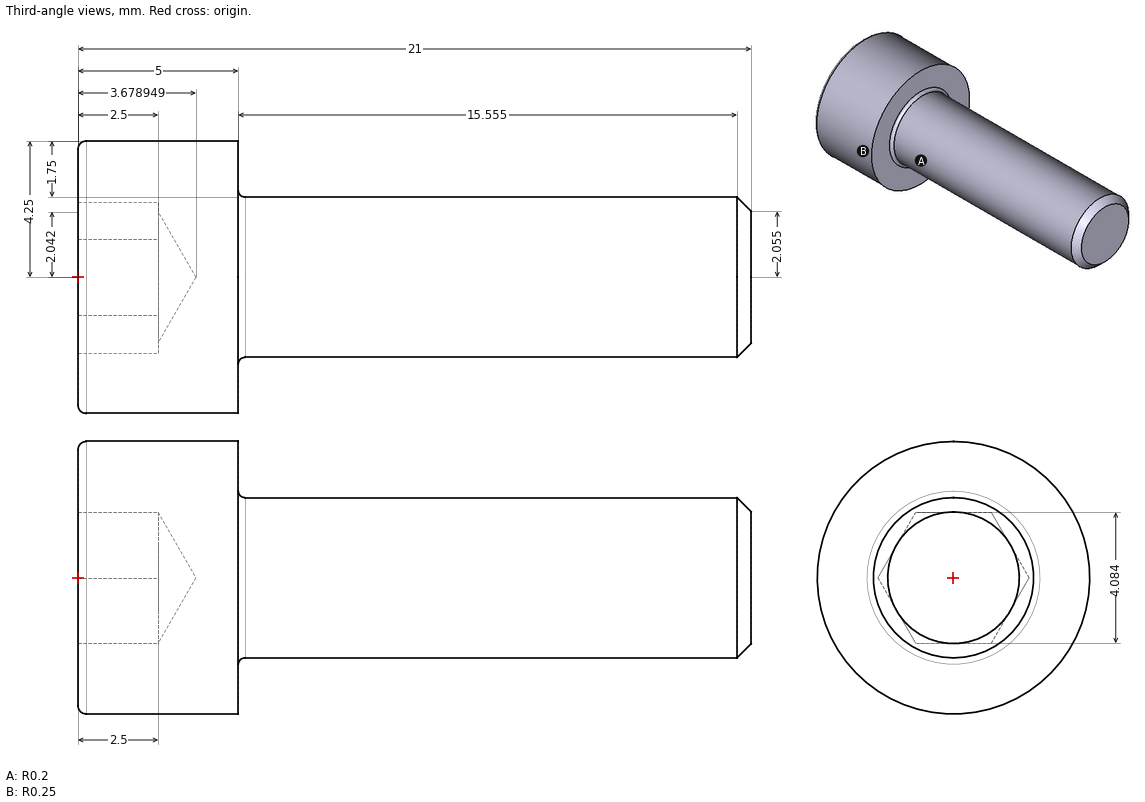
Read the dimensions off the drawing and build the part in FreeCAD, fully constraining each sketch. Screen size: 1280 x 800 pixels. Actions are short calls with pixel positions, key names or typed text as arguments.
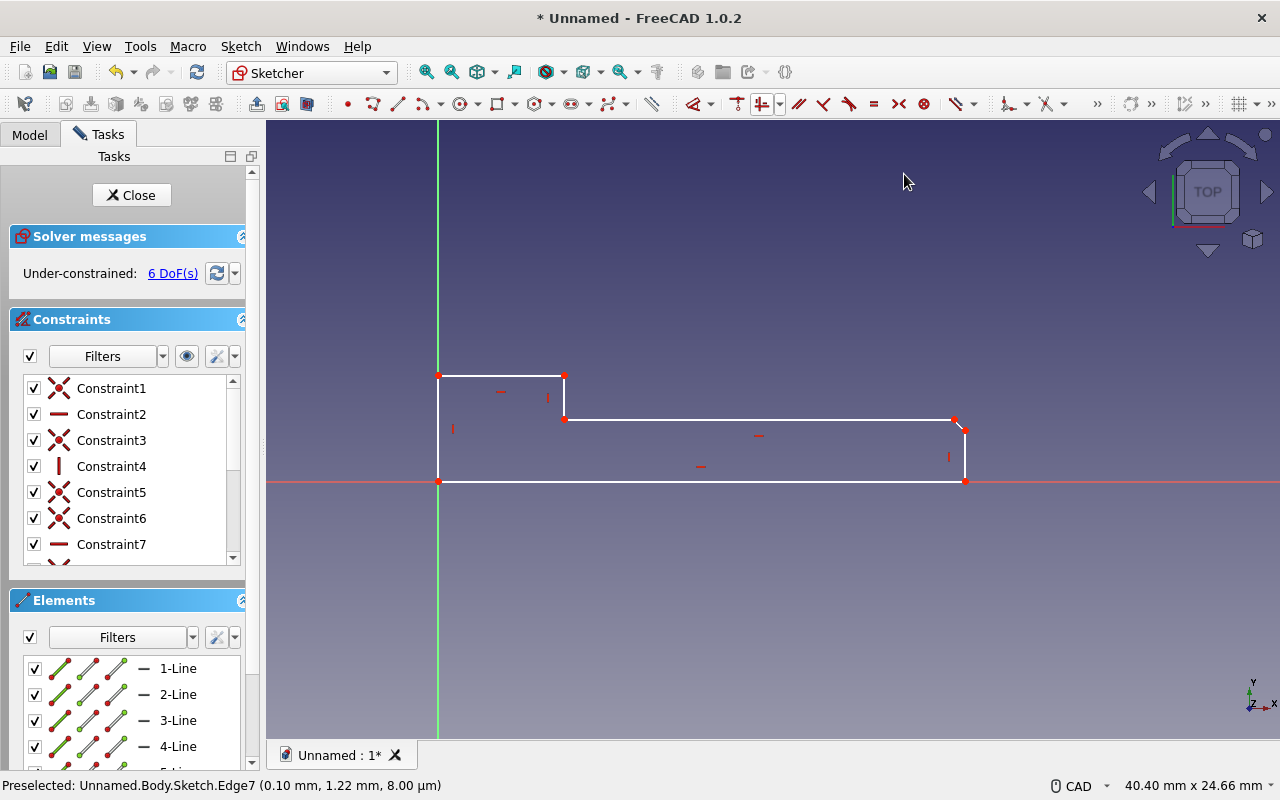
click(692, 104)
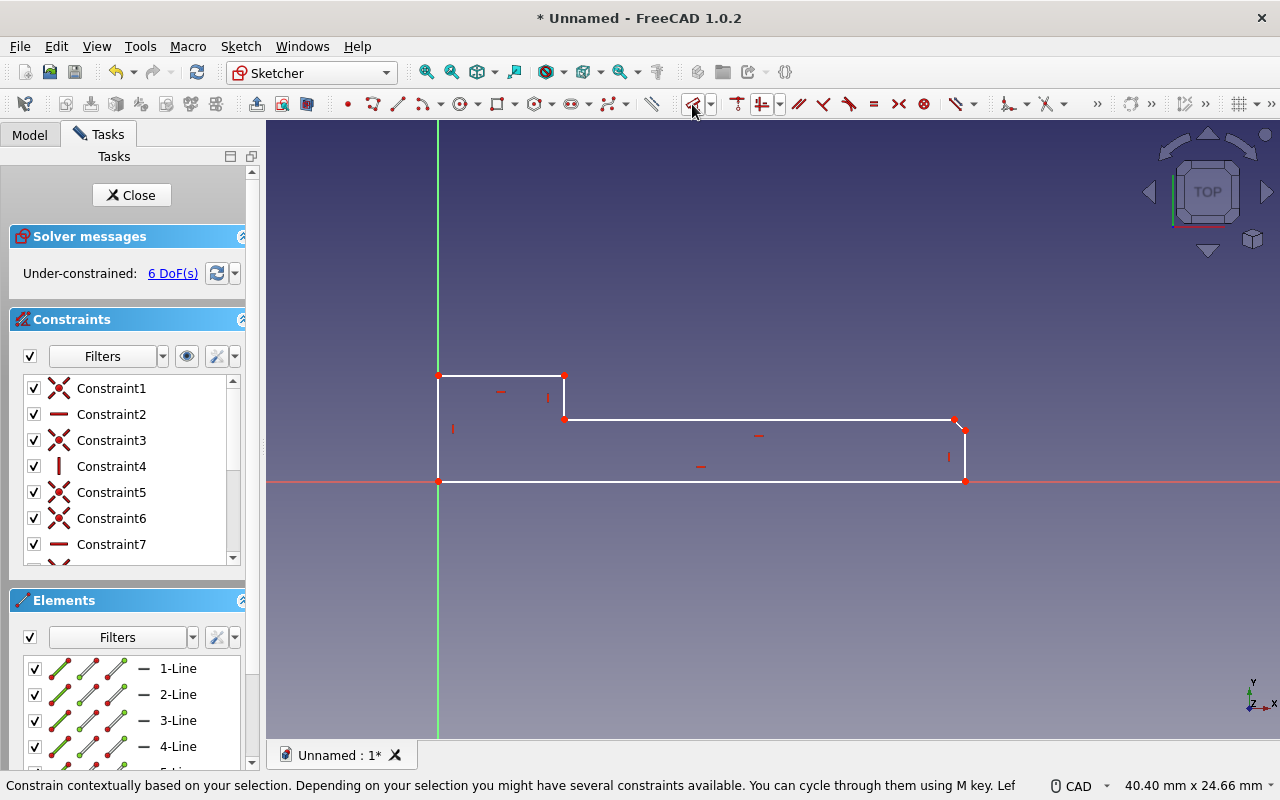
click(526, 376)
click(501, 342)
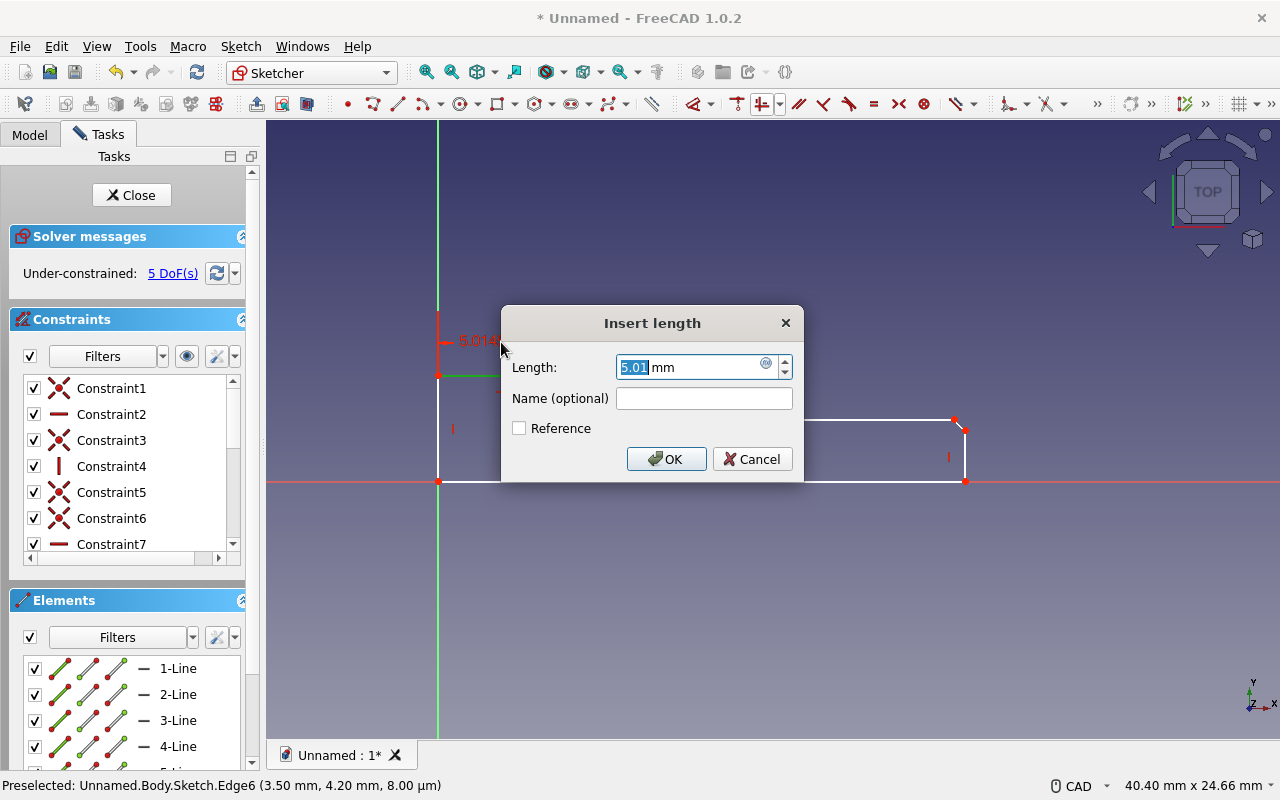
text(5)
key(Return)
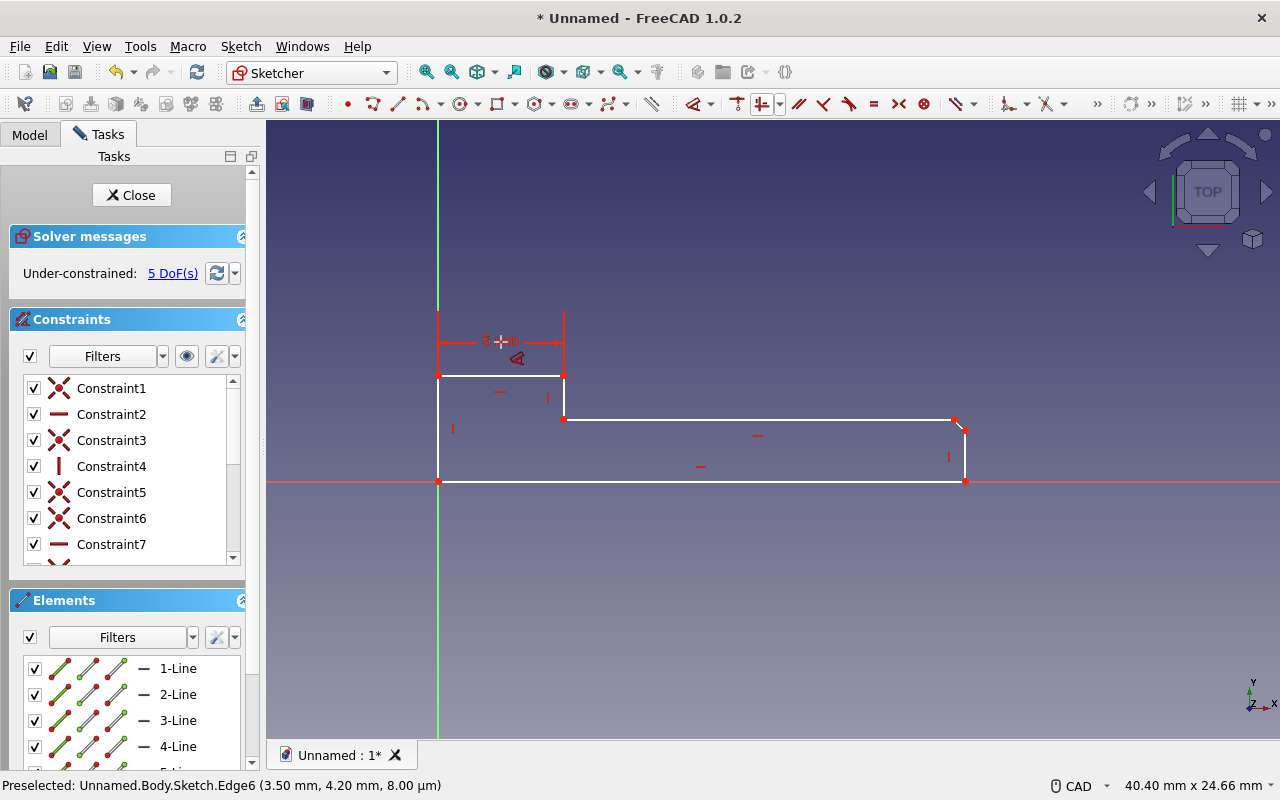
click(596, 482)
click(702, 516)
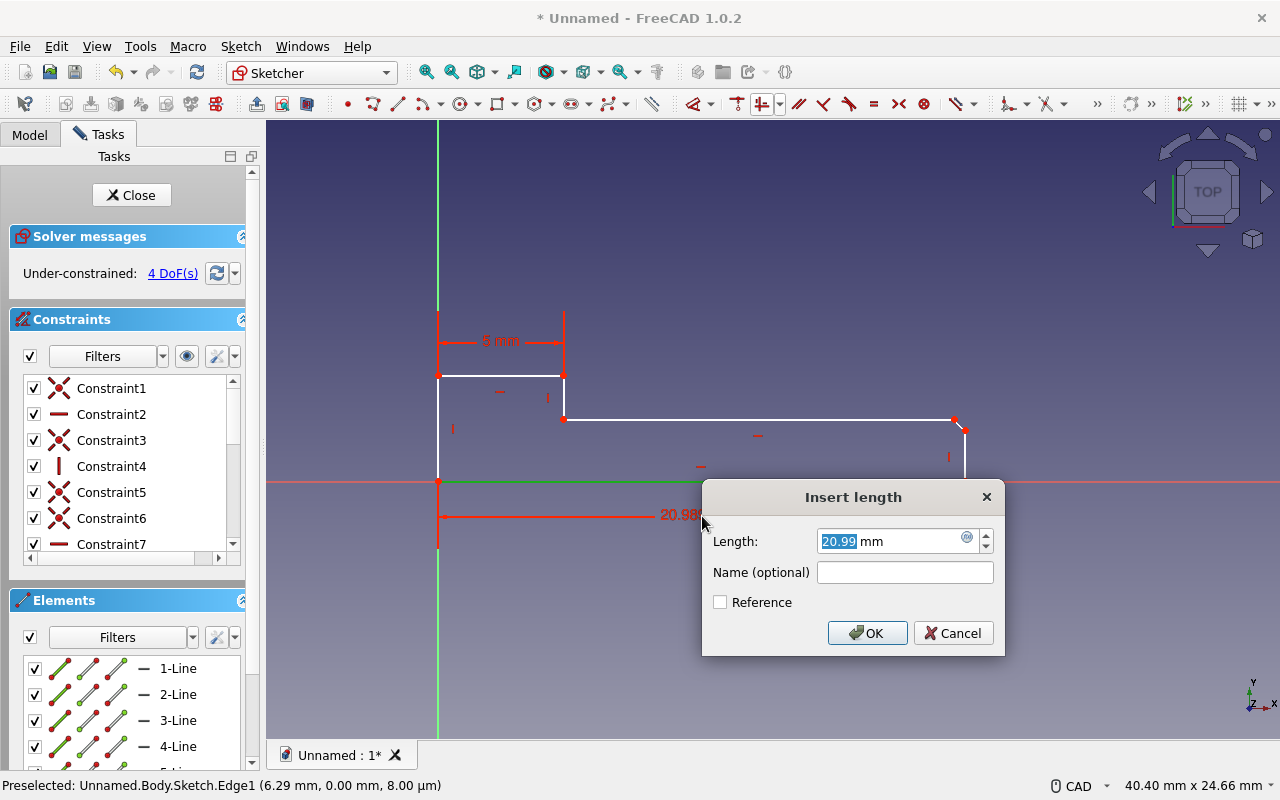
text(21)
key(Return)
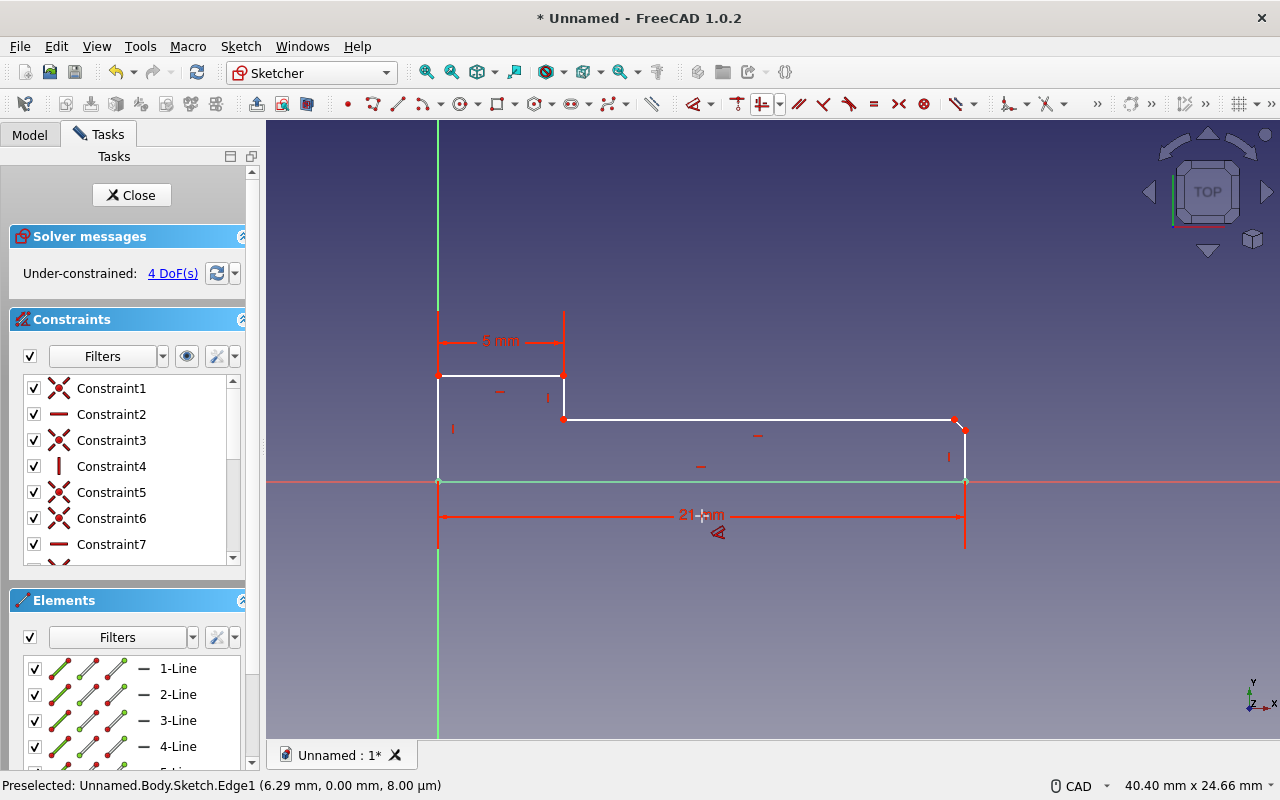
click(564, 407)
click(530, 398)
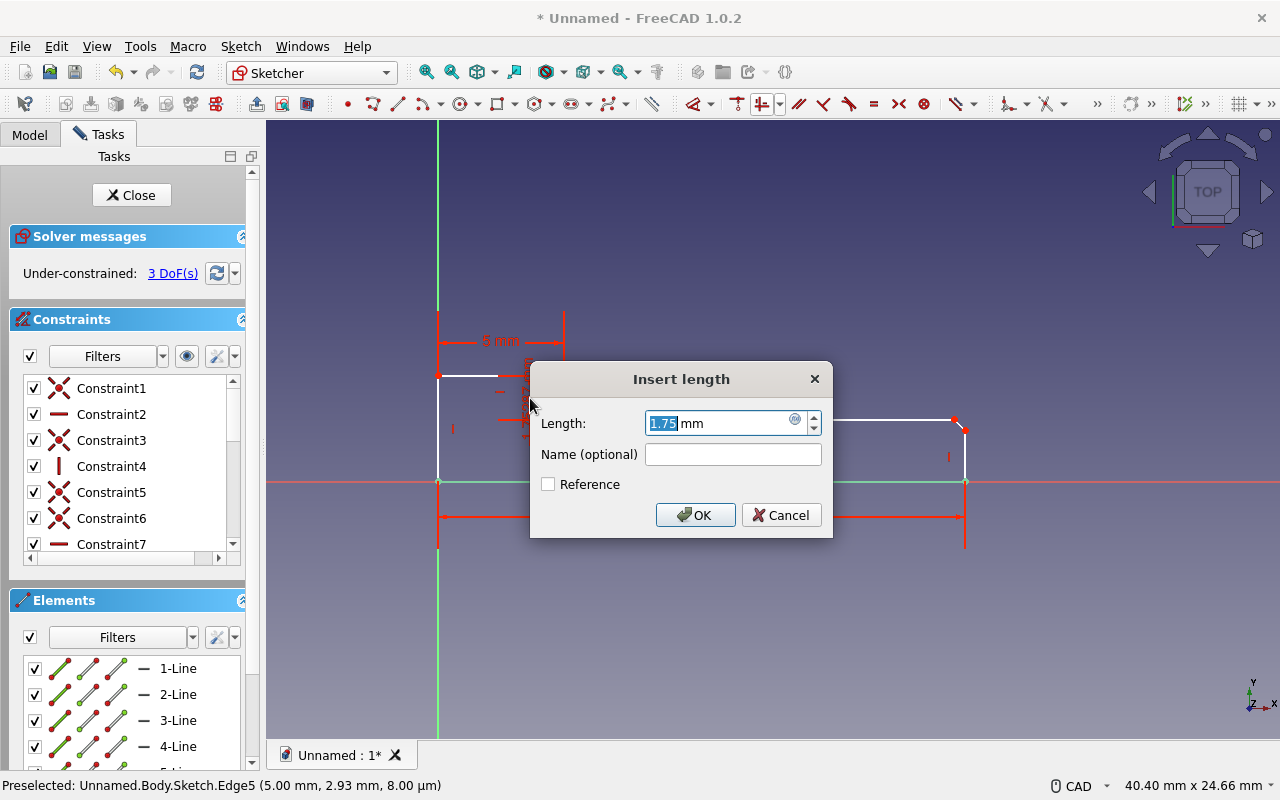
text(1.75)
key(Return)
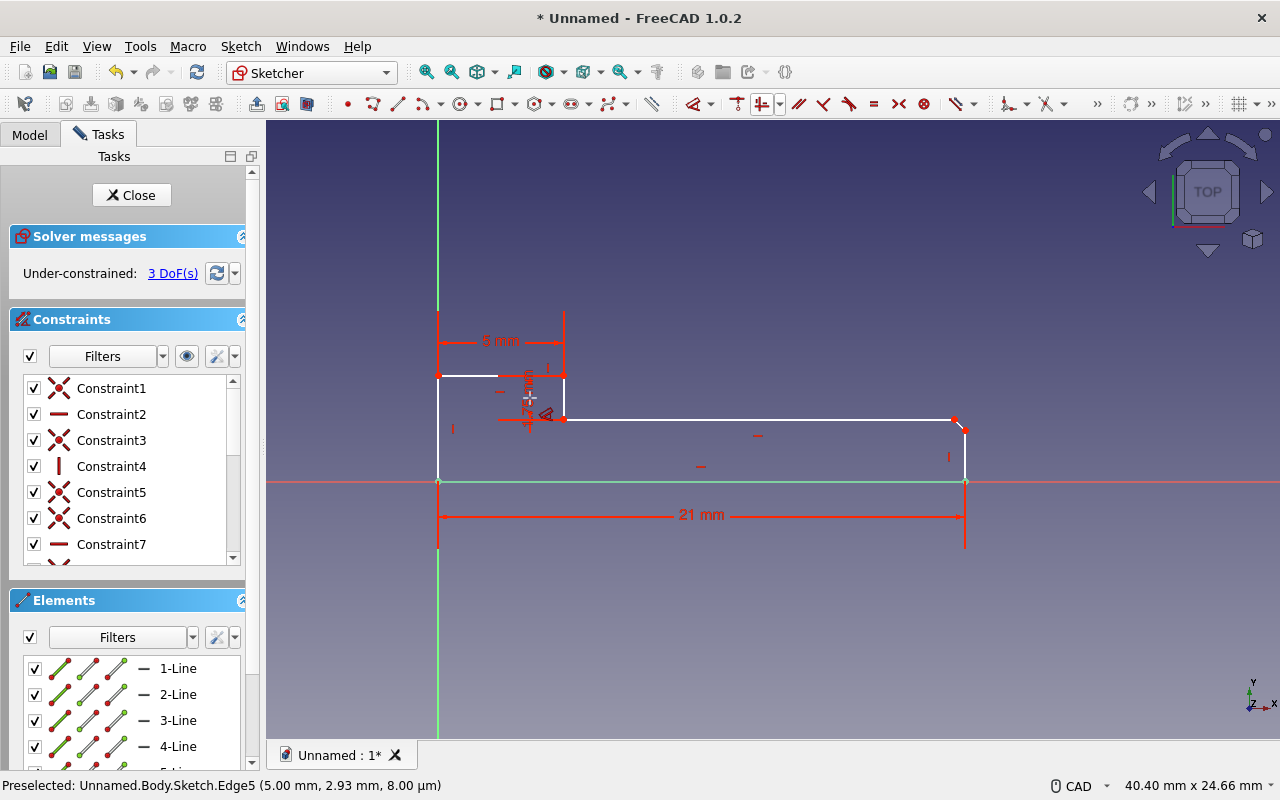
click(438, 408)
click(404, 429)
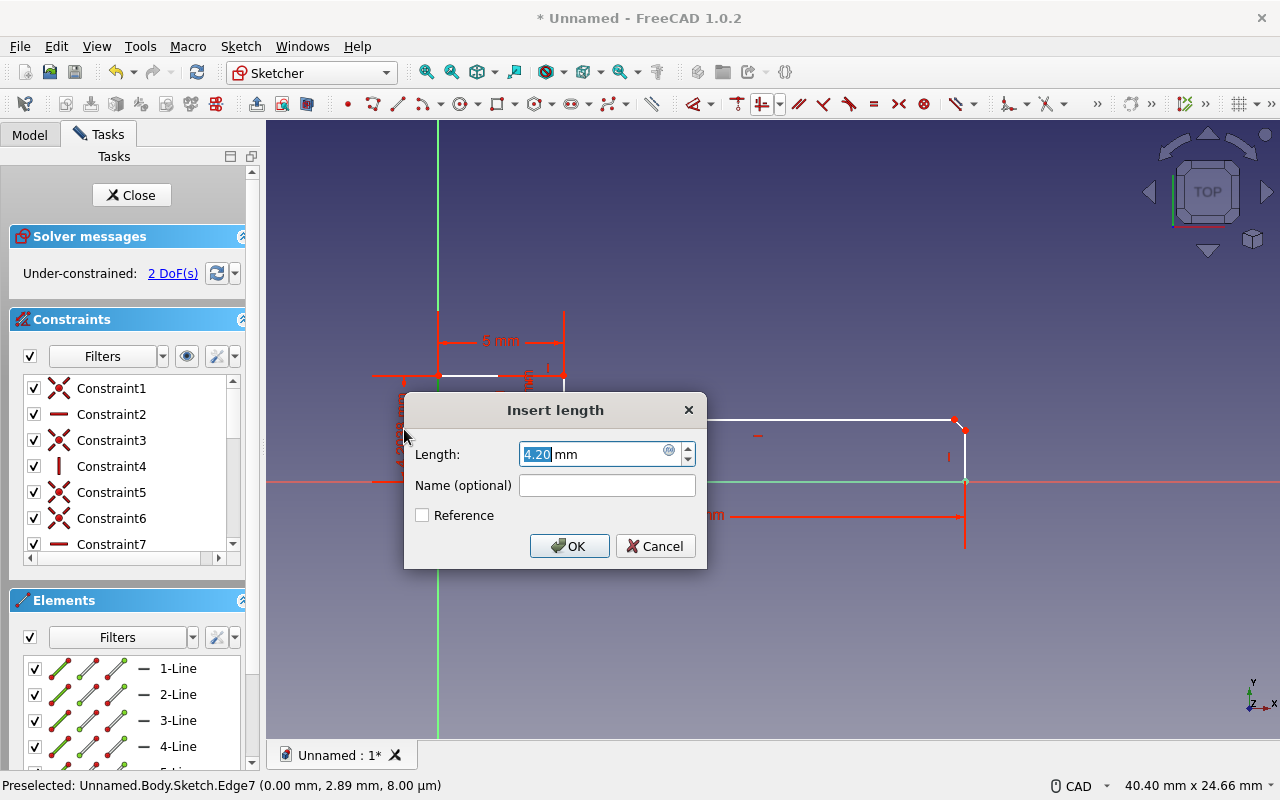
text(4.25)
key(Return)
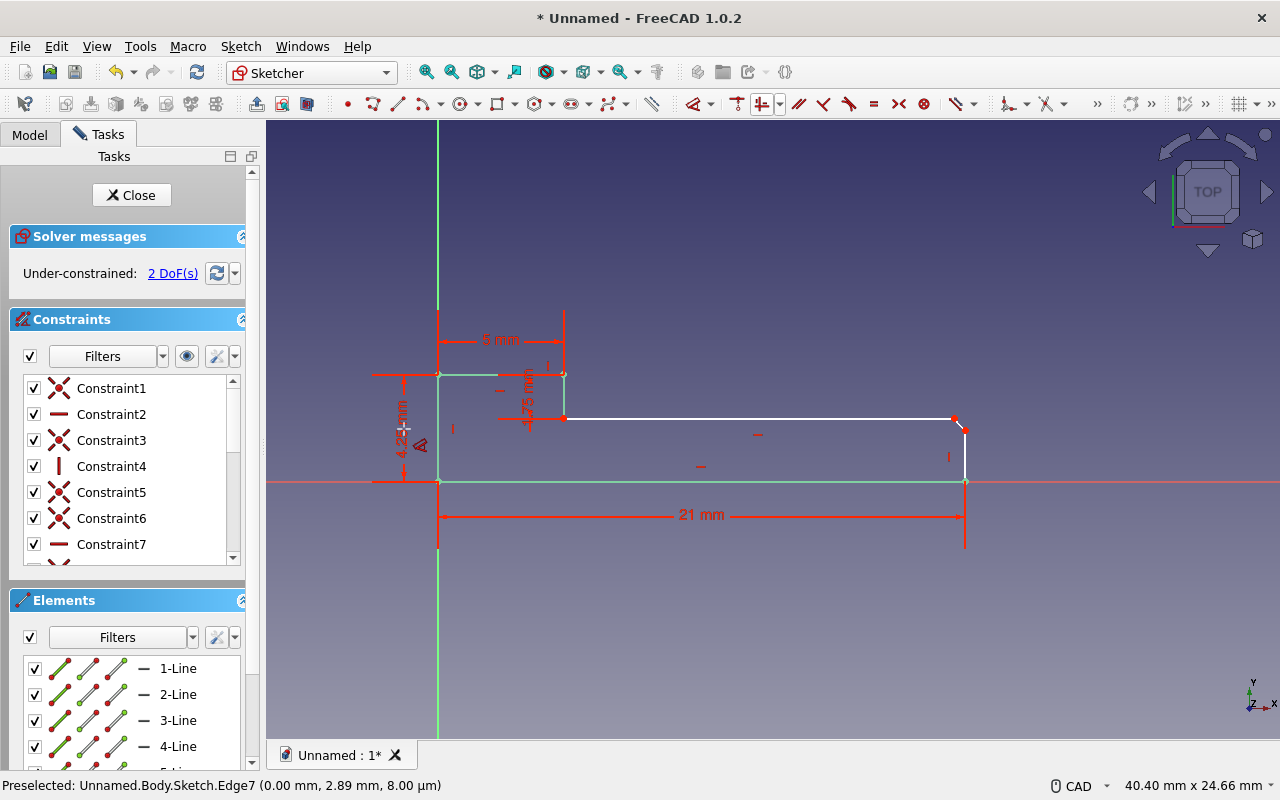
click(965, 466)
click(999, 456)